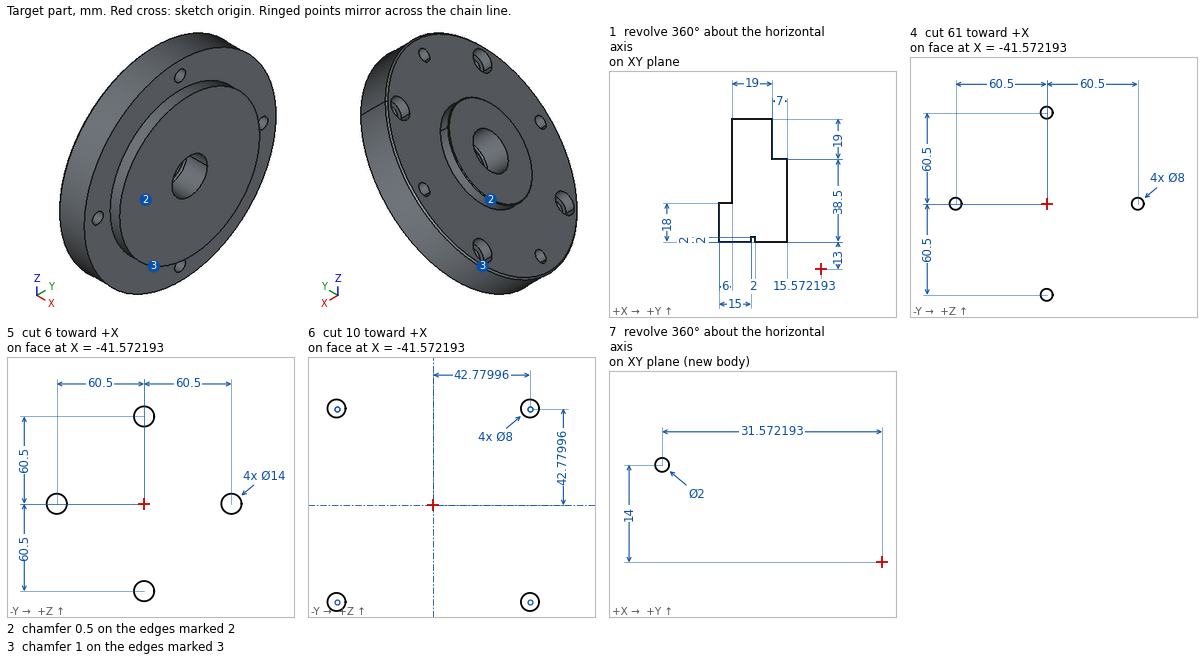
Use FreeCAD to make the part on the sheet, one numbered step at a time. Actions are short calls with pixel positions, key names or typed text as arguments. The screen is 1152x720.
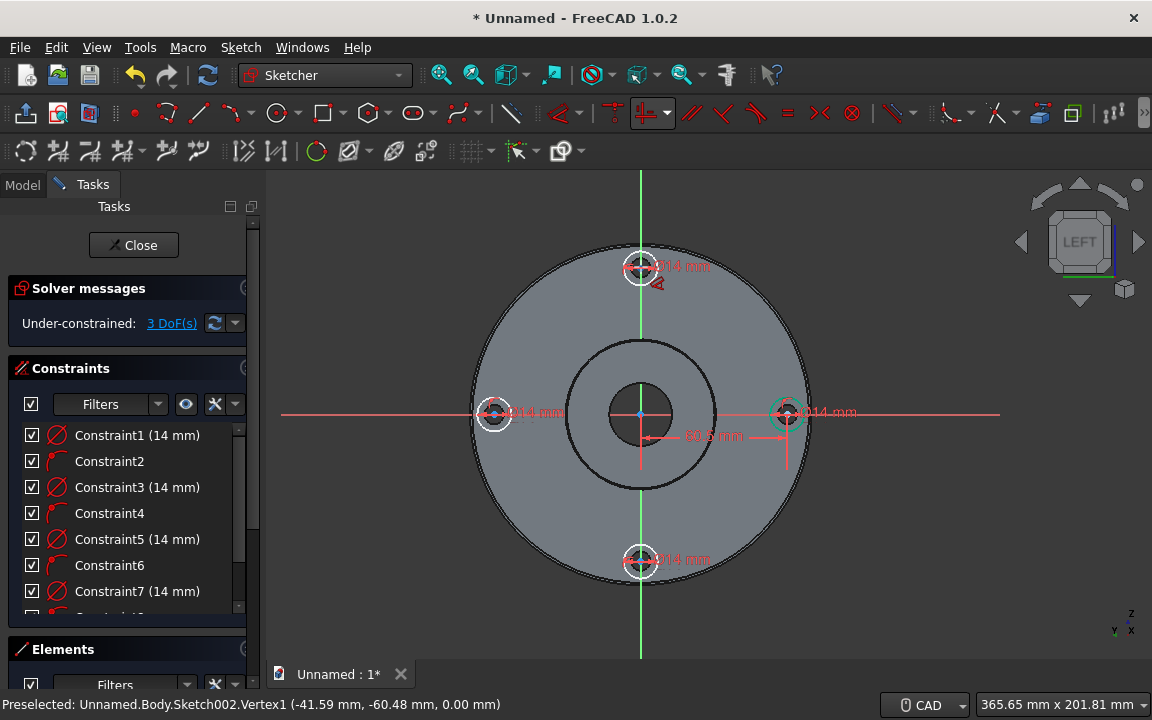
click(641, 562)
click(675, 488)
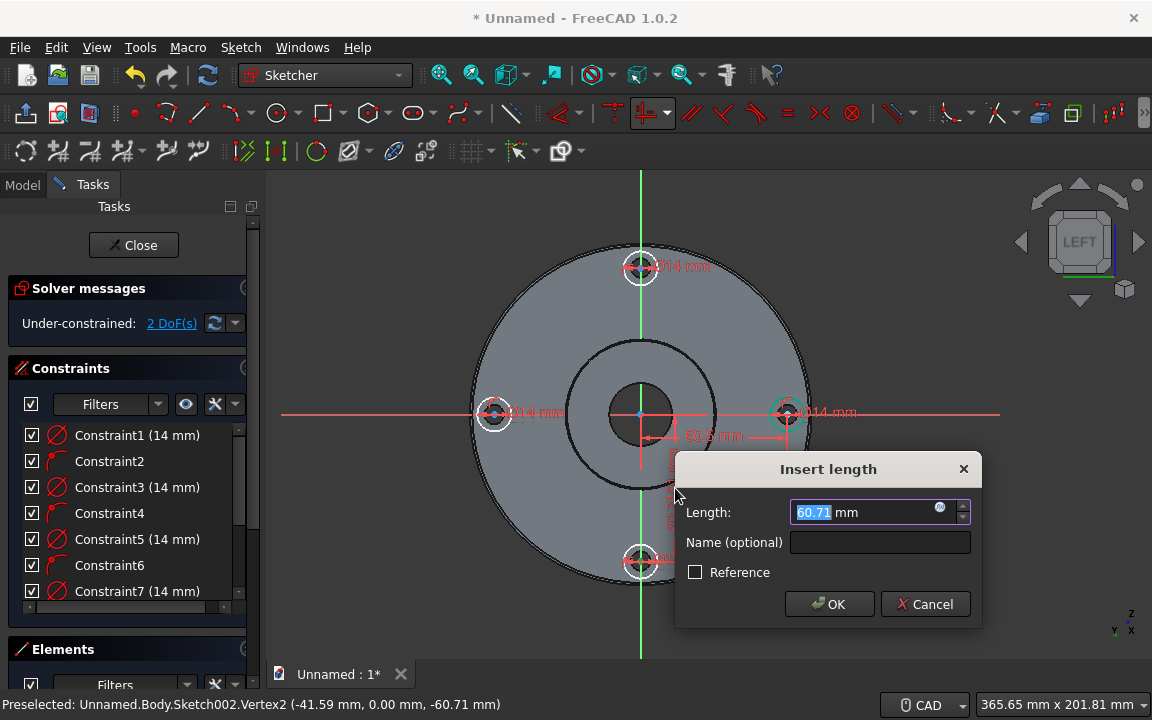
text(60.5)
key(Return)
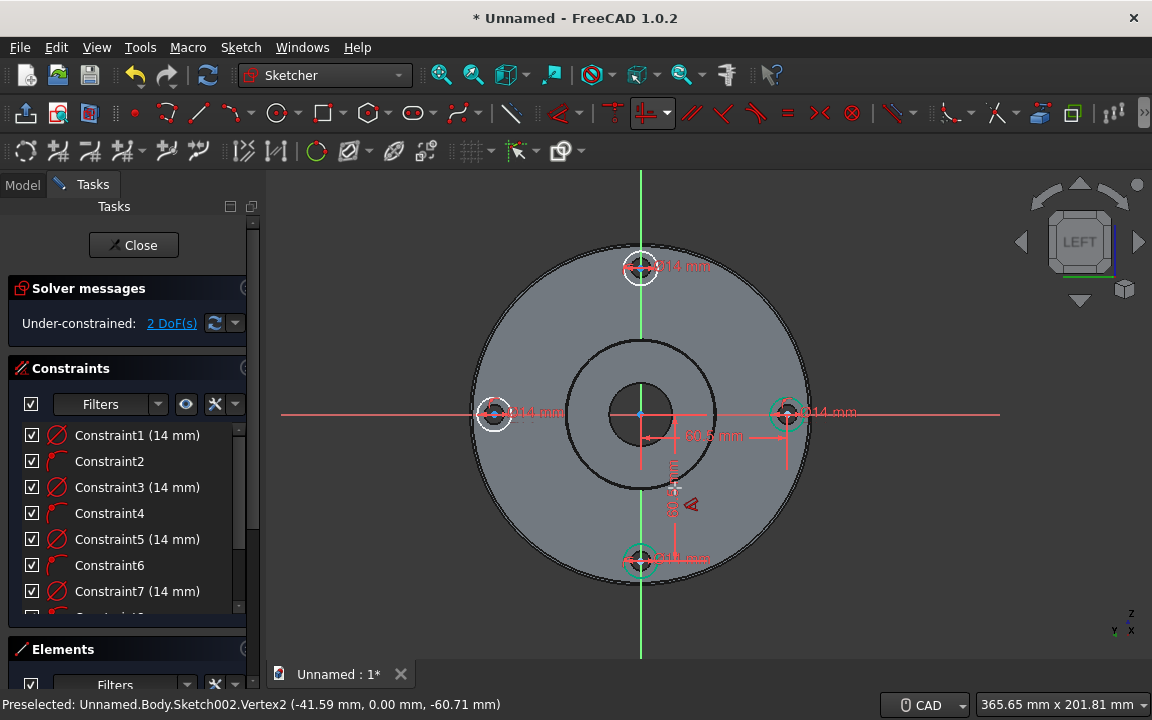
click(641, 268)
click(675, 341)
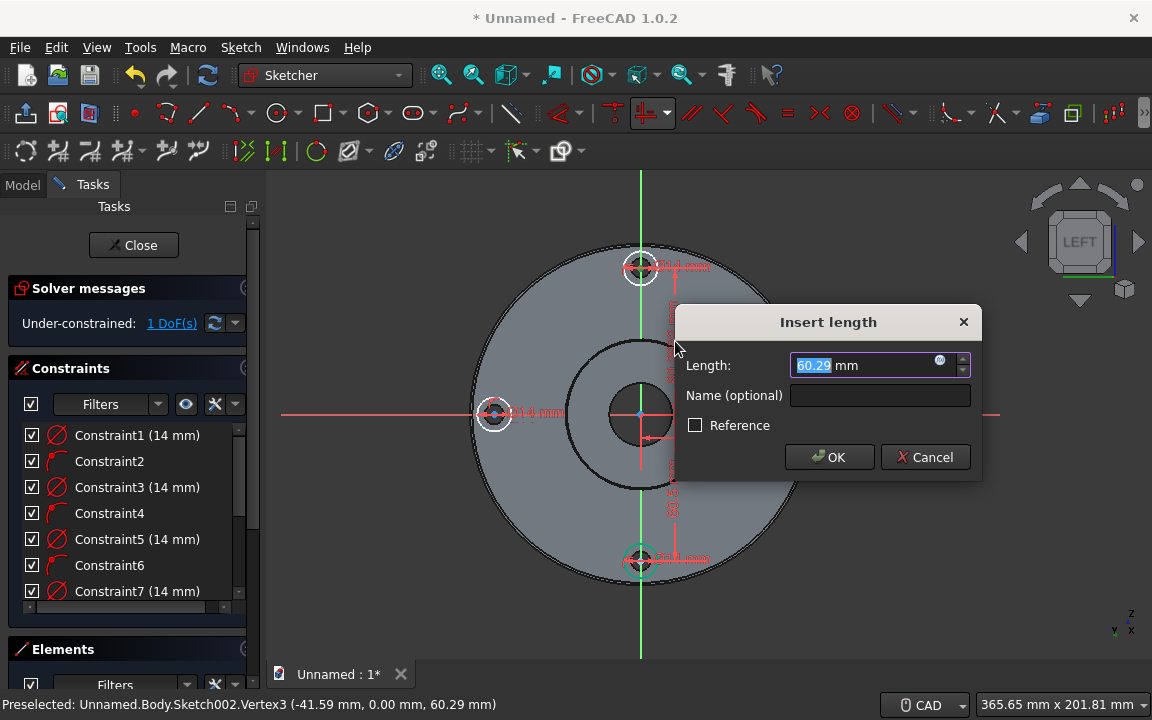
text(60.5)
key(Return)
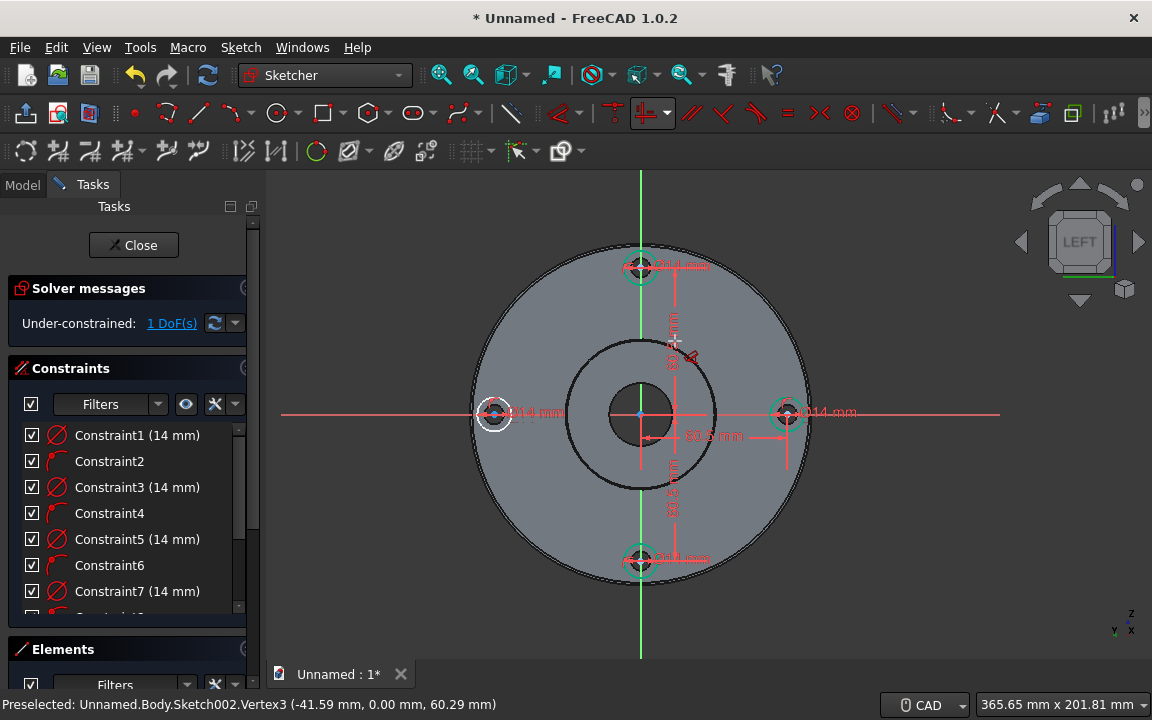
click(494, 415)
click(568, 449)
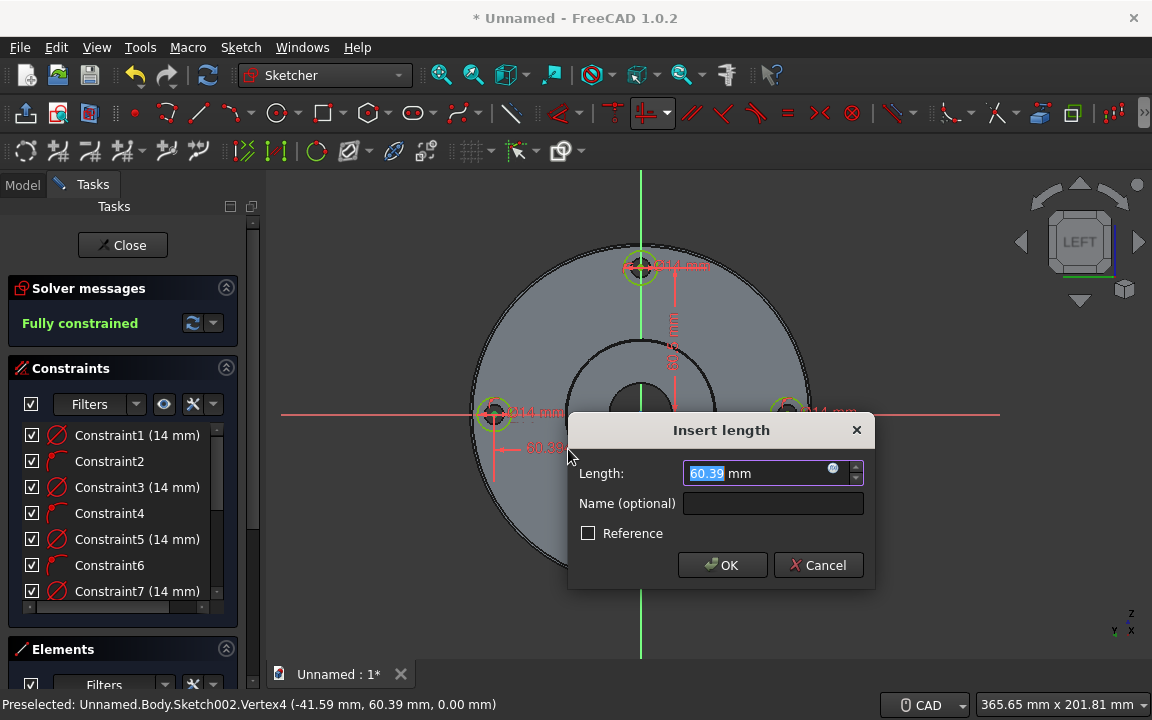
text(60.5)
key(Return)
key(Escape)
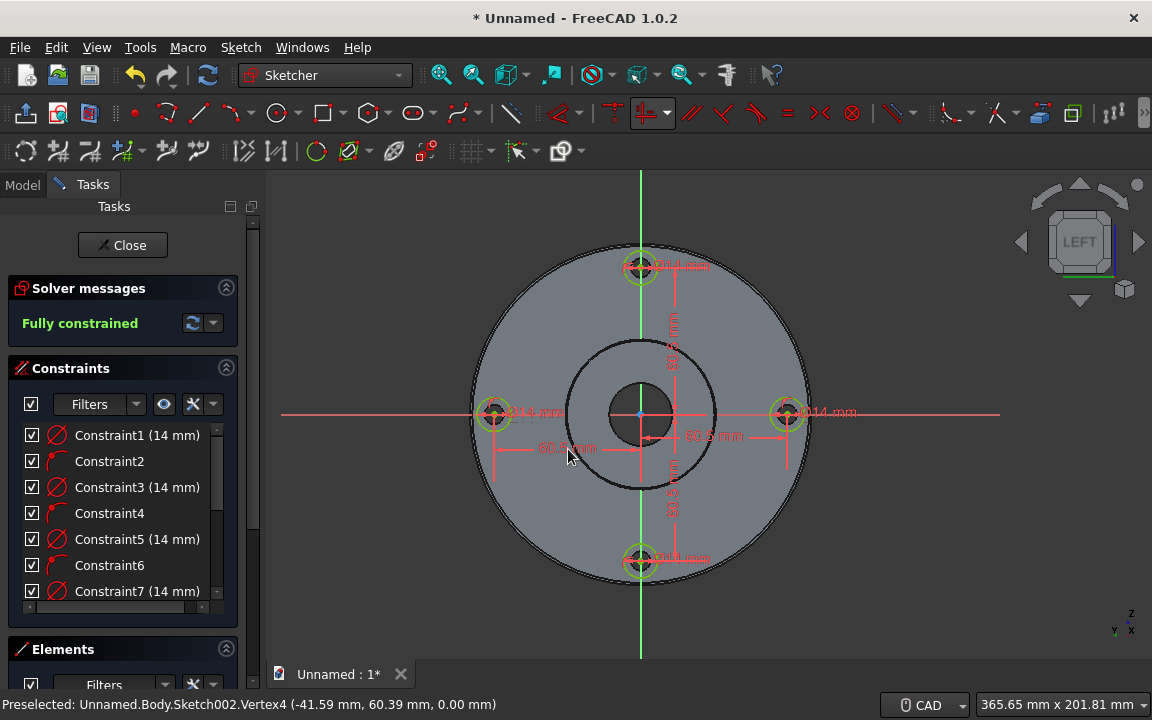
click(123, 245)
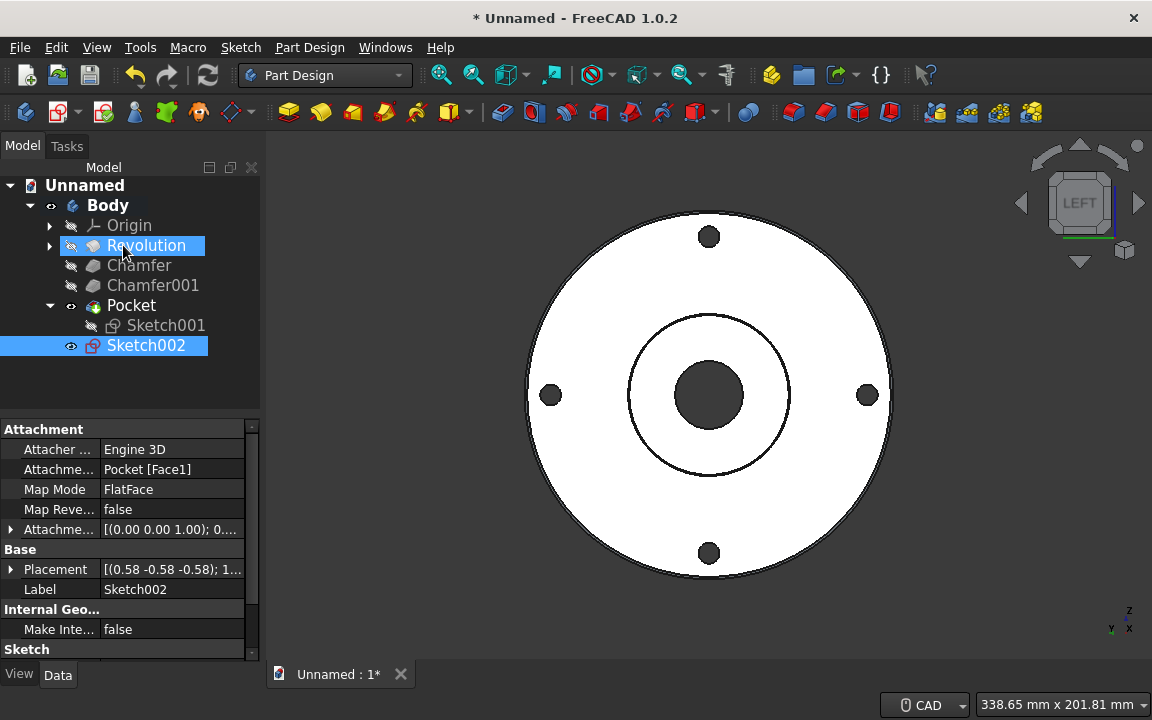
click(504, 112)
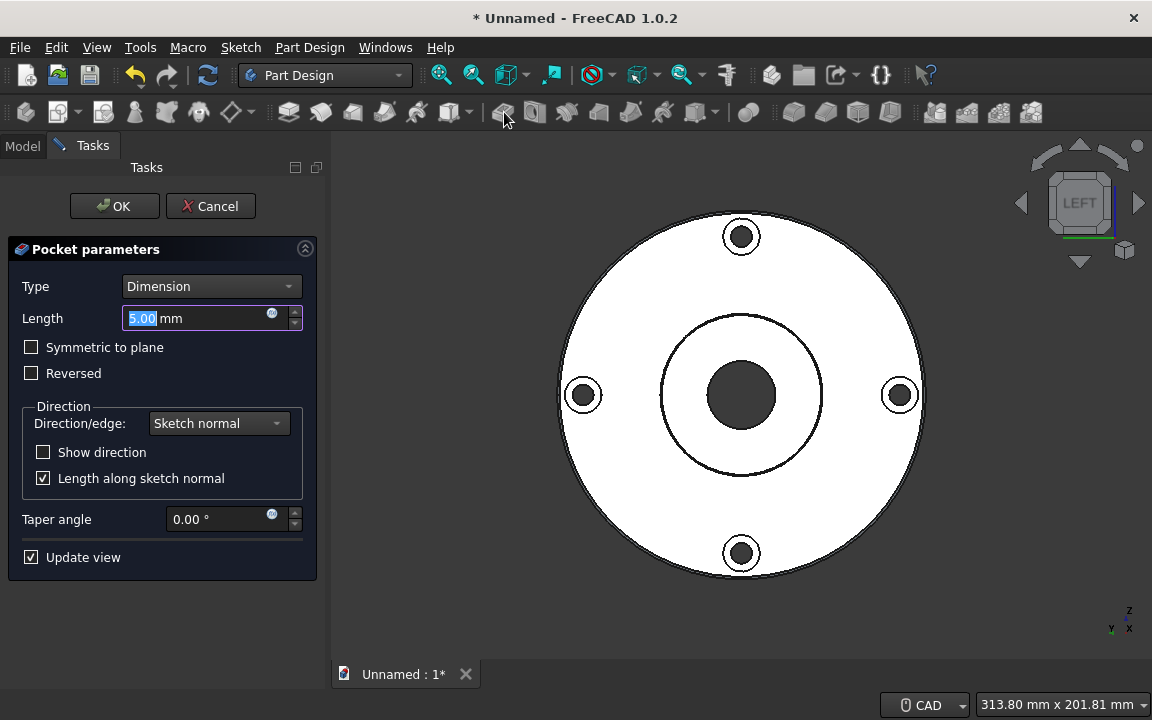
text(6)
key(Tab)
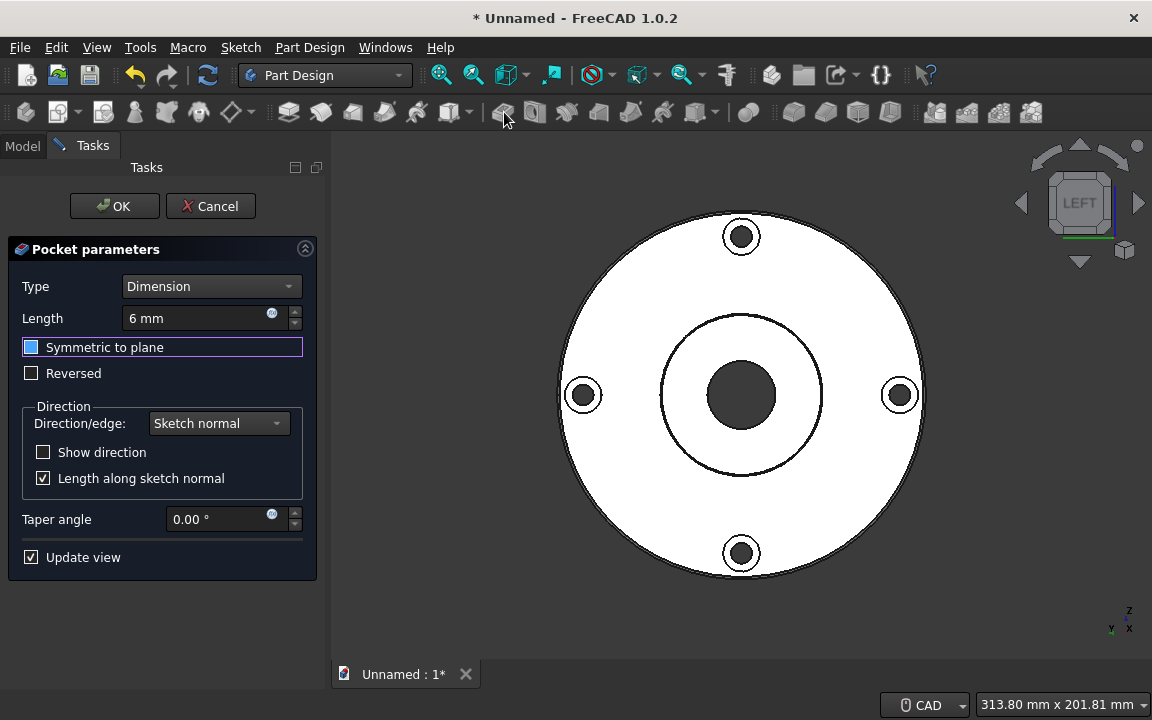
click(115, 206)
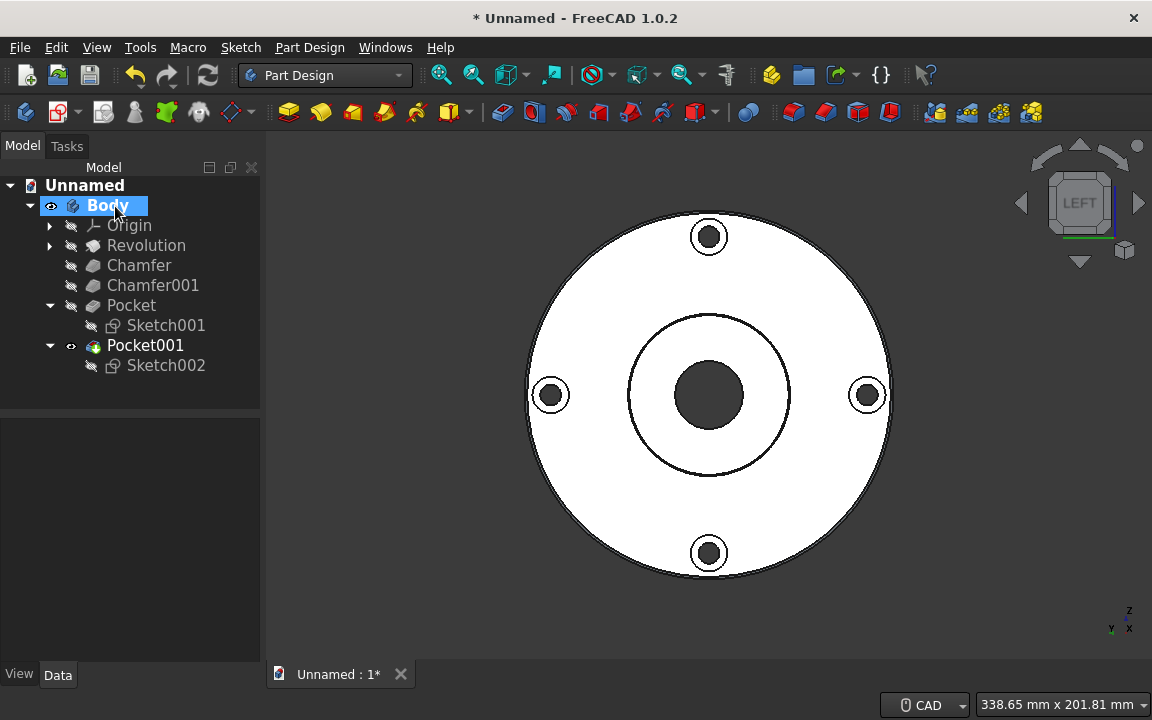
click(657, 498)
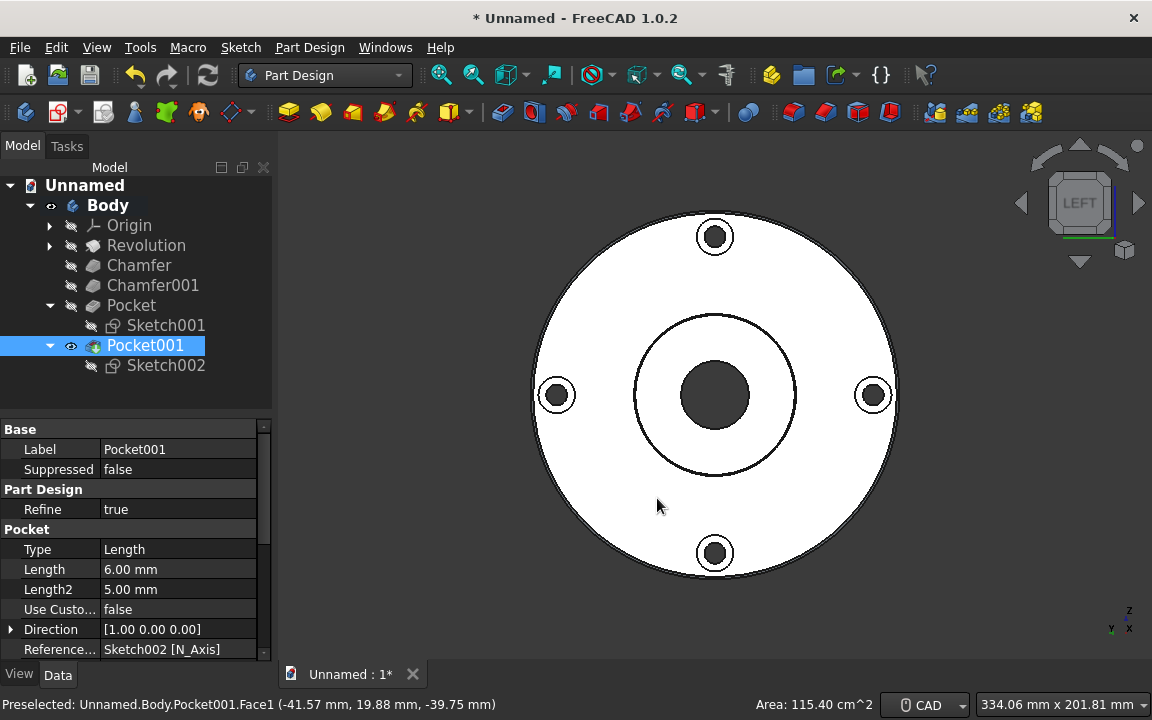
click(58, 112)